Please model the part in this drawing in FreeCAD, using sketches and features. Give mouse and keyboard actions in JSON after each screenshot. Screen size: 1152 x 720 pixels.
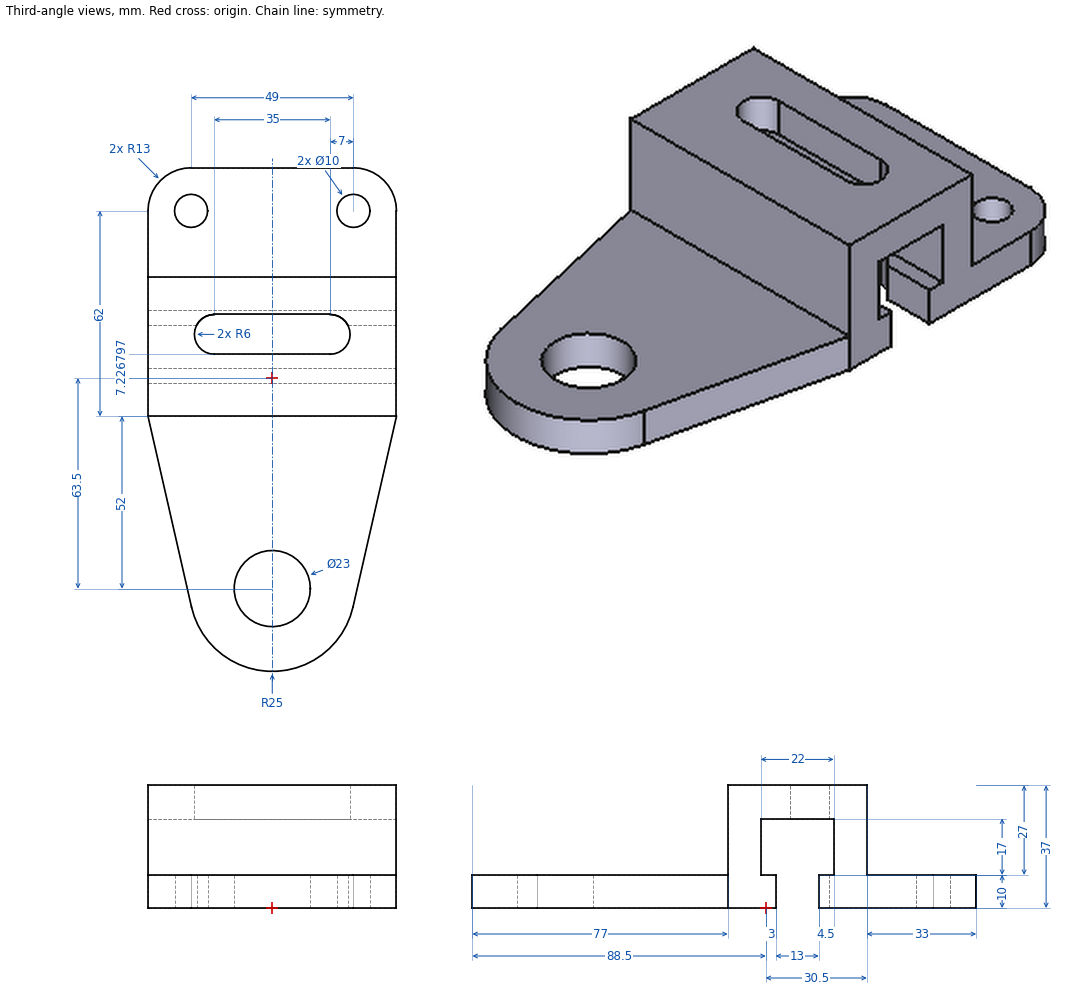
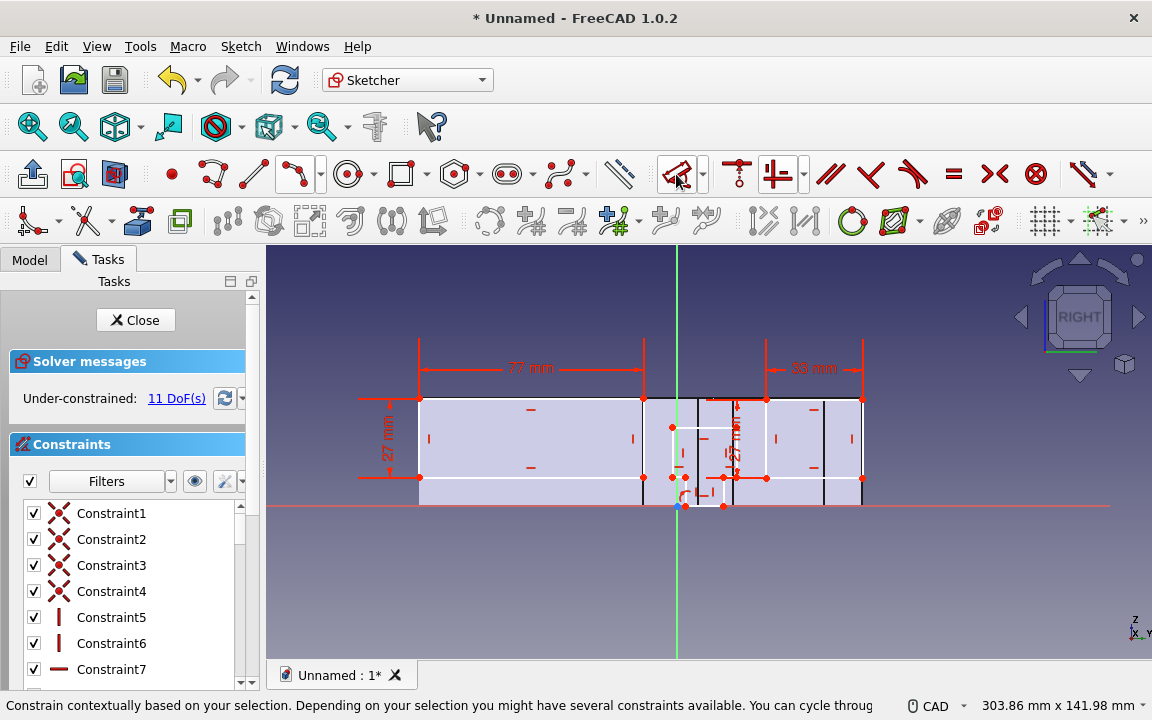
{"action": "left_click", "coordinate": [697, 506]}
{"action": "left_click", "coordinate": [705, 540]}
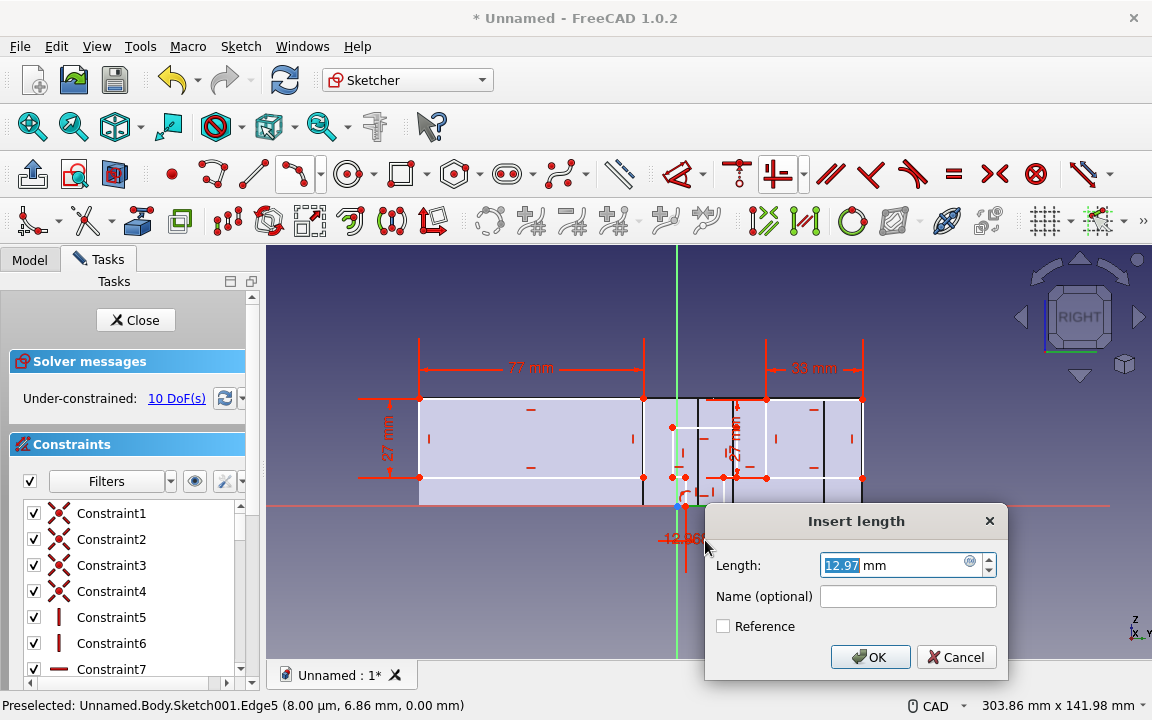
{"action": "type", "text": "13"}
{"action": "key", "text": "Return"}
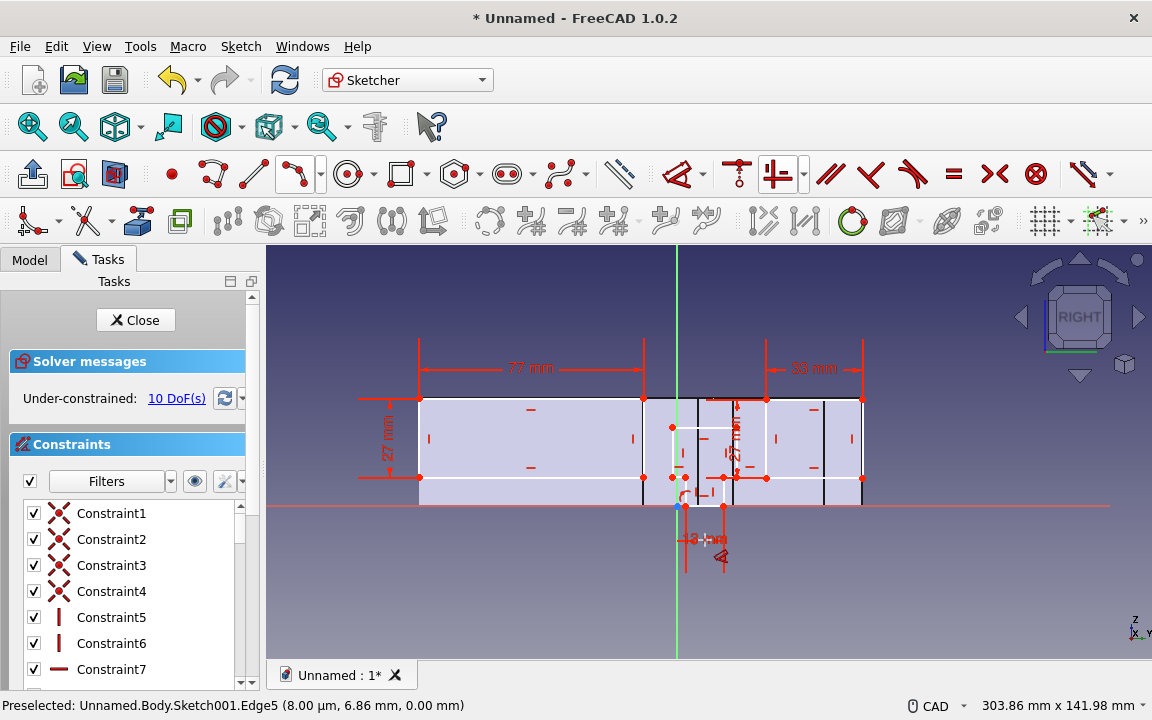
{"action": "scroll", "coordinate": [724, 494], "scroll_direction": "up", "scroll_amount": 2}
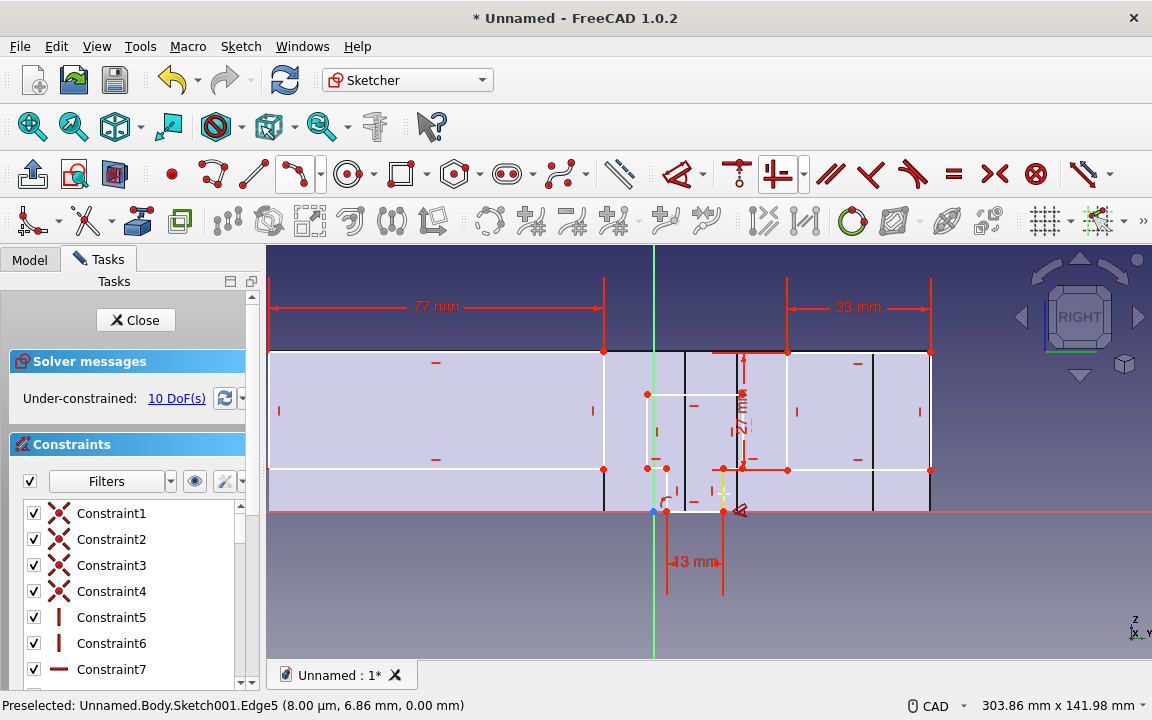
{"action": "left_click", "coordinate": [723, 494]}
{"action": "left_click", "coordinate": [757, 490]}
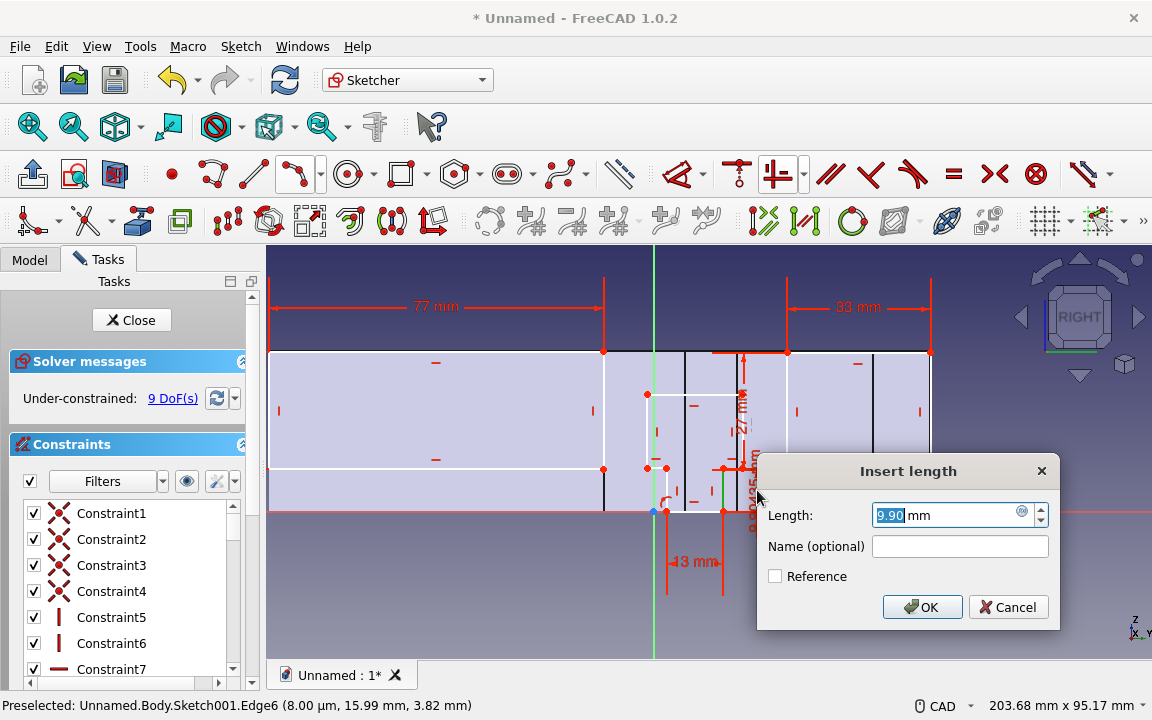
{"action": "type", "text": "10"}
{"action": "key", "text": "Return"}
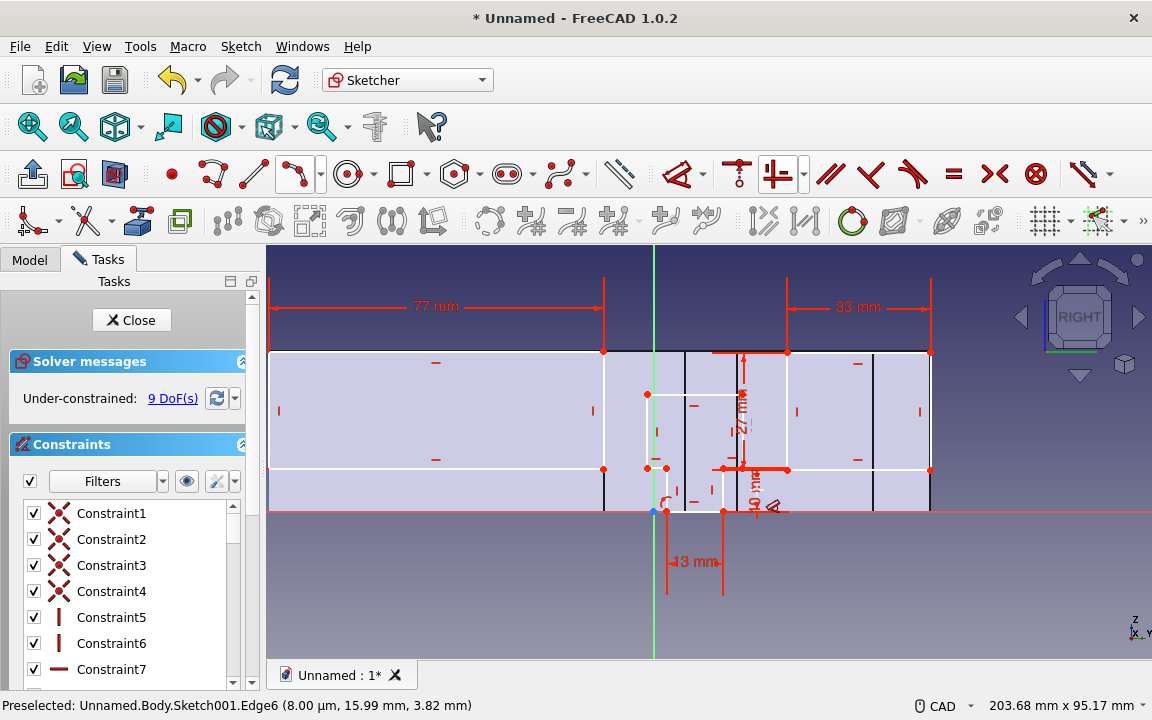
{"action": "left_click", "coordinate": [743, 446]}
{"action": "left_click", "coordinate": [709, 431]}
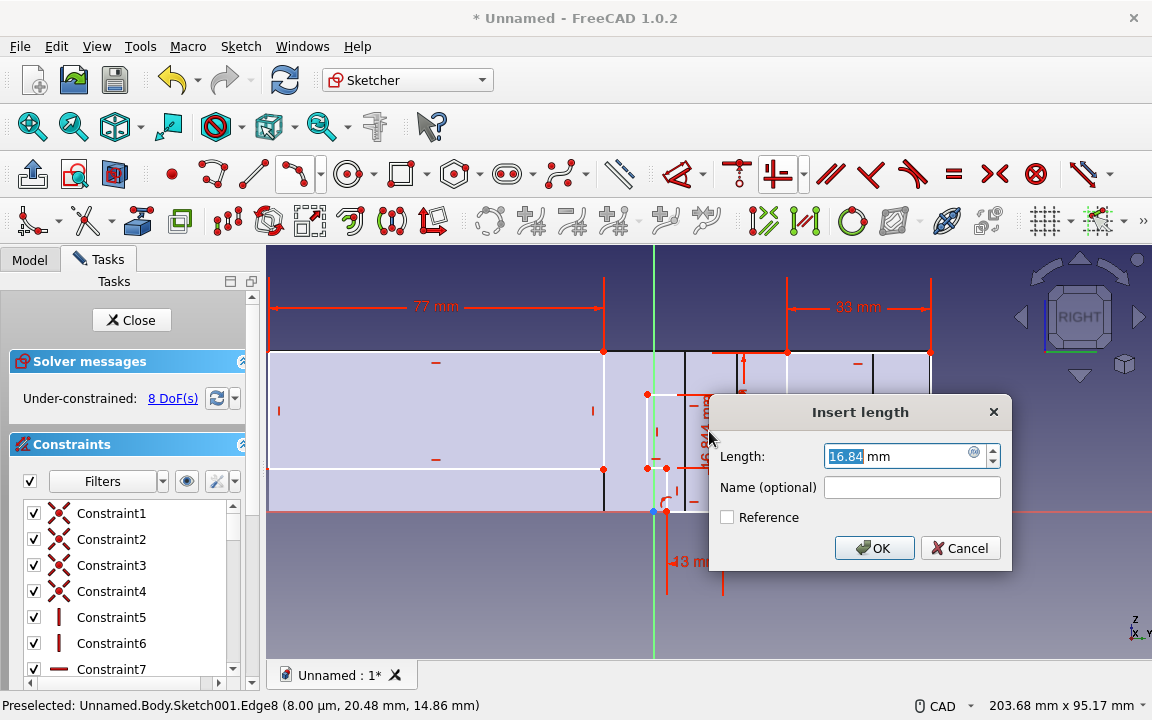
{"action": "type", "text": "17"}
{"action": "key", "text": "Return"}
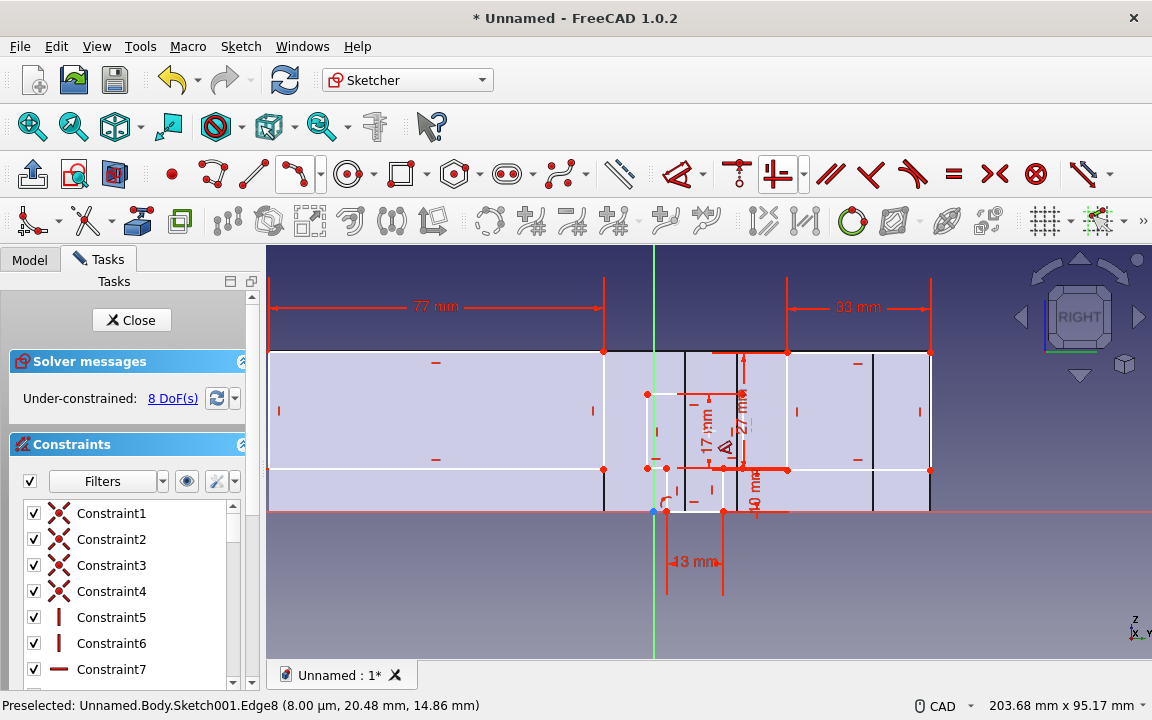
{"action": "left_click", "coordinate": [714, 394]}
{"action": "left_click", "coordinate": [695, 360]}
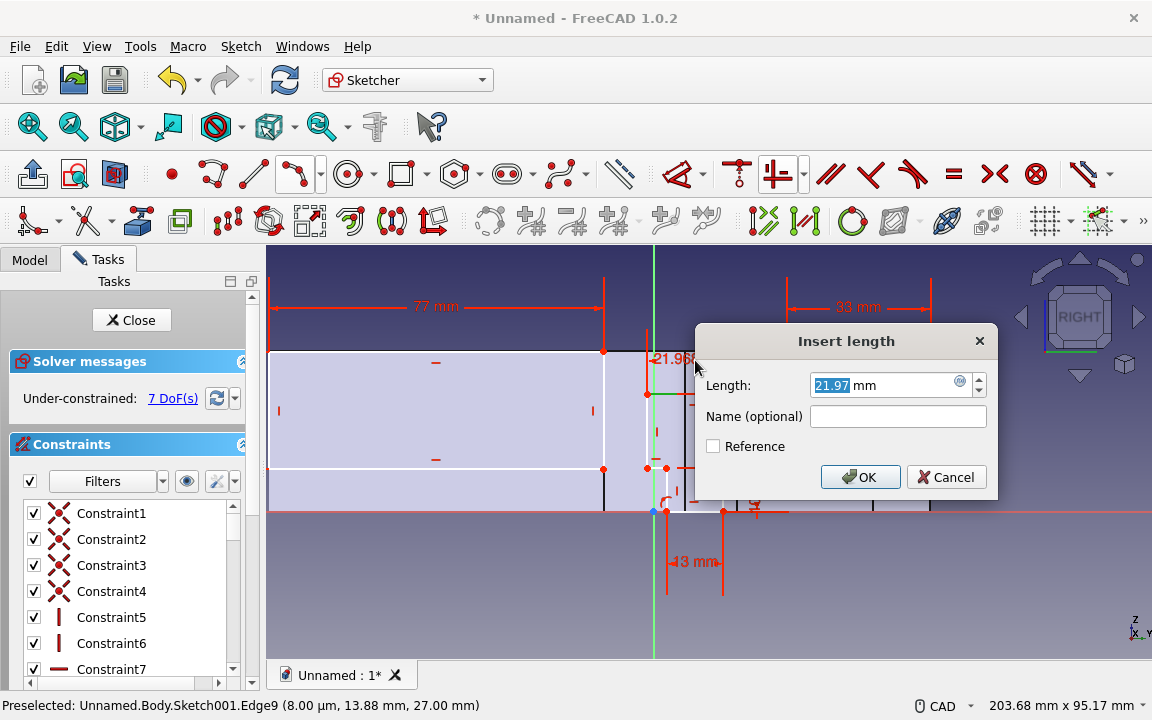
{"action": "type", "text": "22"}
{"action": "key", "text": "Return"}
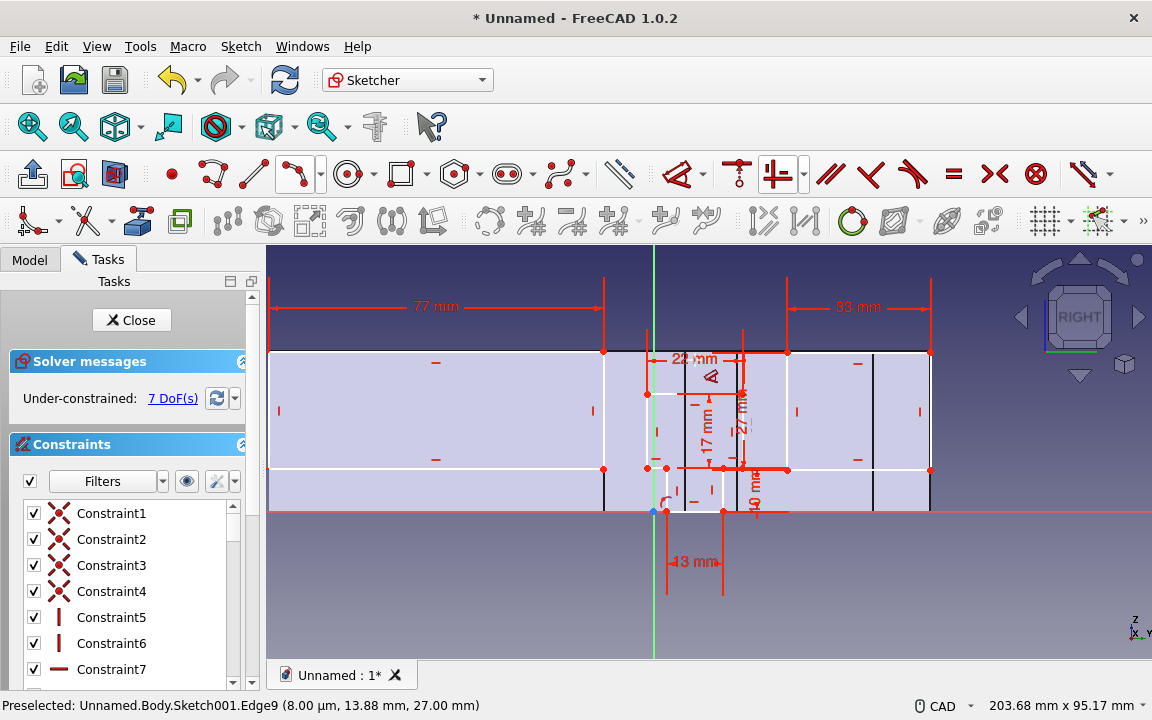
{"action": "scroll", "coordinate": [647, 416], "scroll_direction": "up", "scroll_amount": 4}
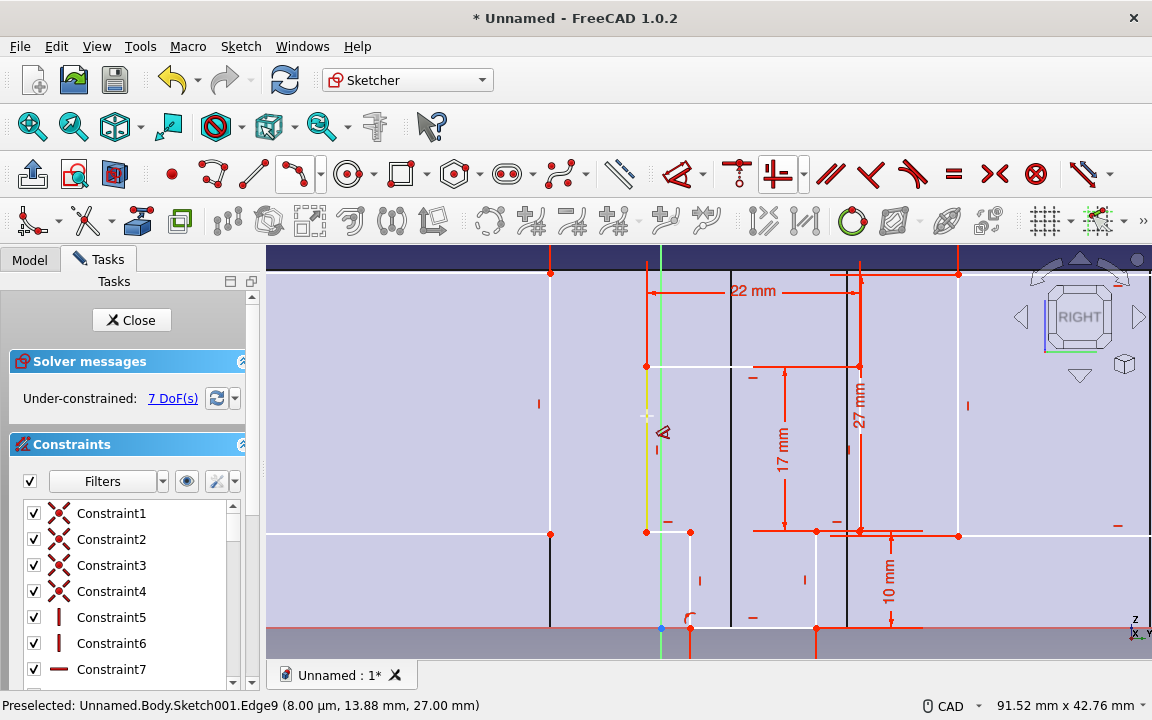
{"action": "left_click", "coordinate": [647, 417]}
{"action": "left_click", "coordinate": [681, 450]}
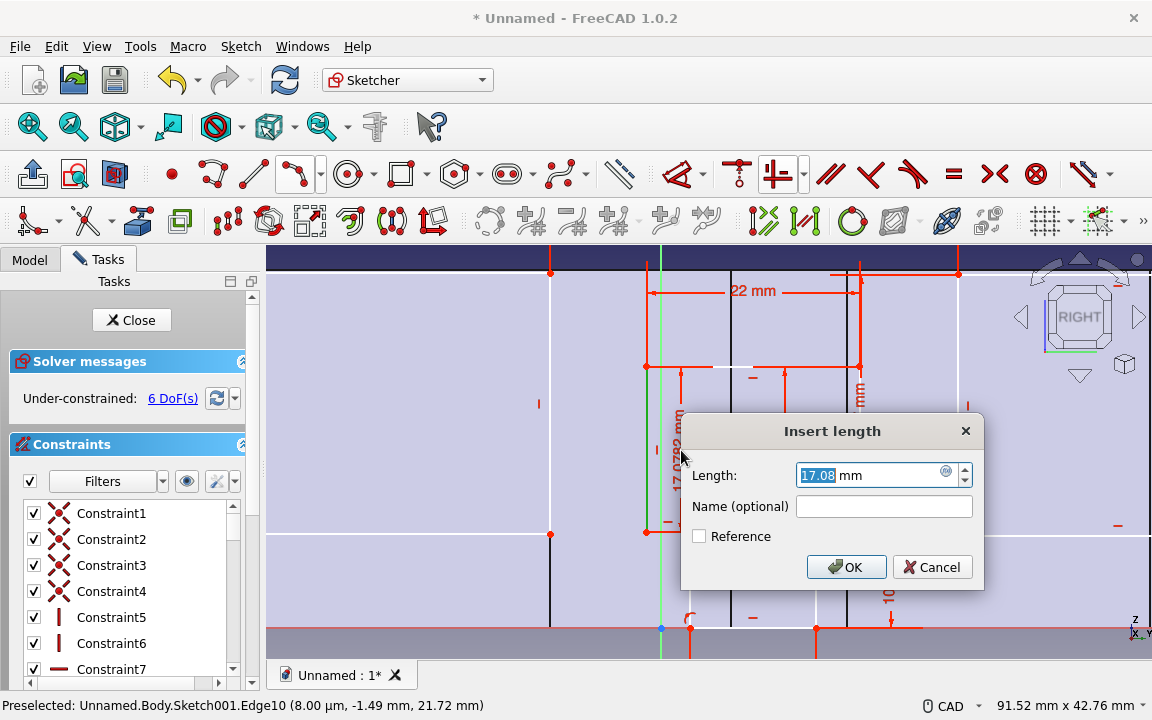
{"action": "type", "text": "17"}
{"action": "key", "text": "Return"}